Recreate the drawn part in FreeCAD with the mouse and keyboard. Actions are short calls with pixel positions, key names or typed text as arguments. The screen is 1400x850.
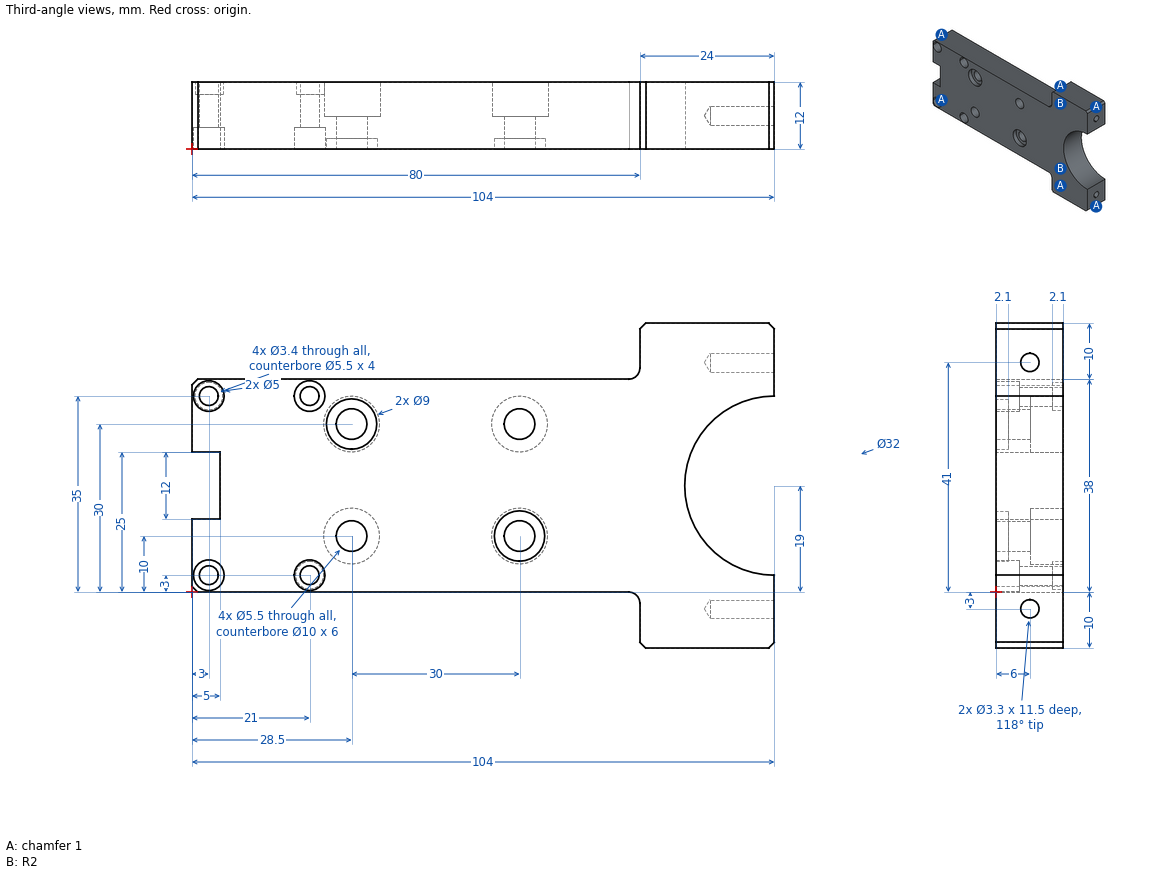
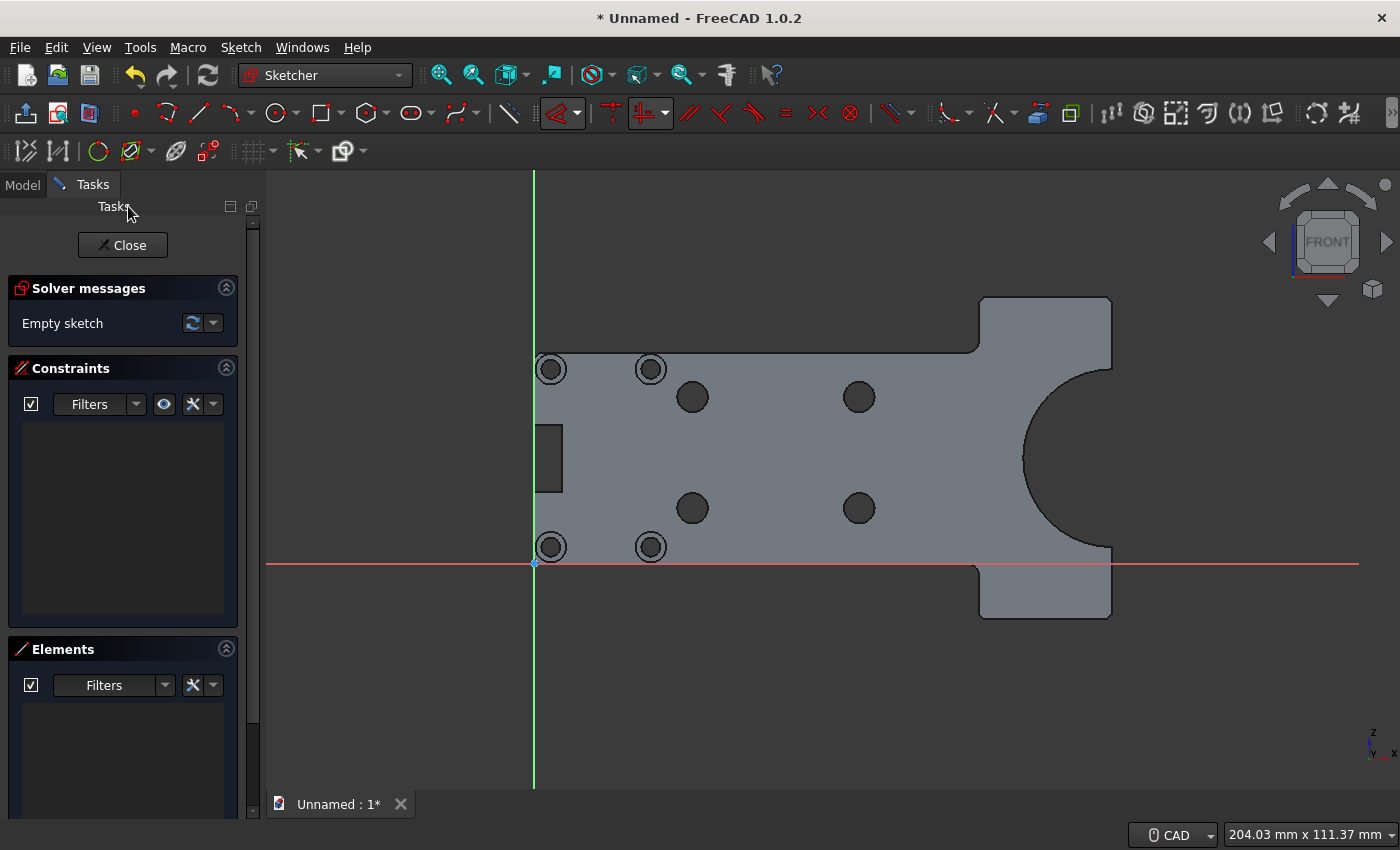
scroll(642, 454, up, 3)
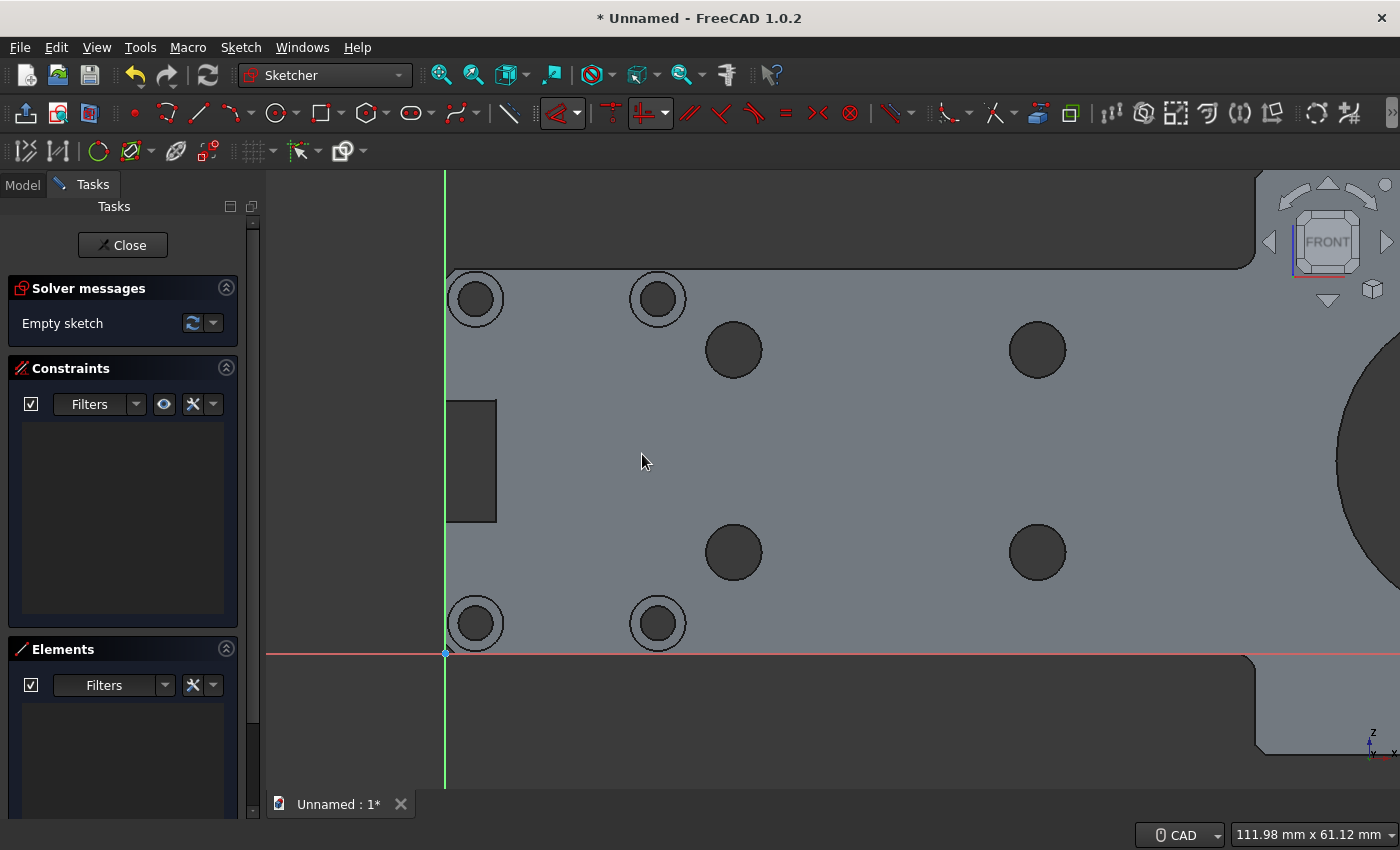
click(276, 114)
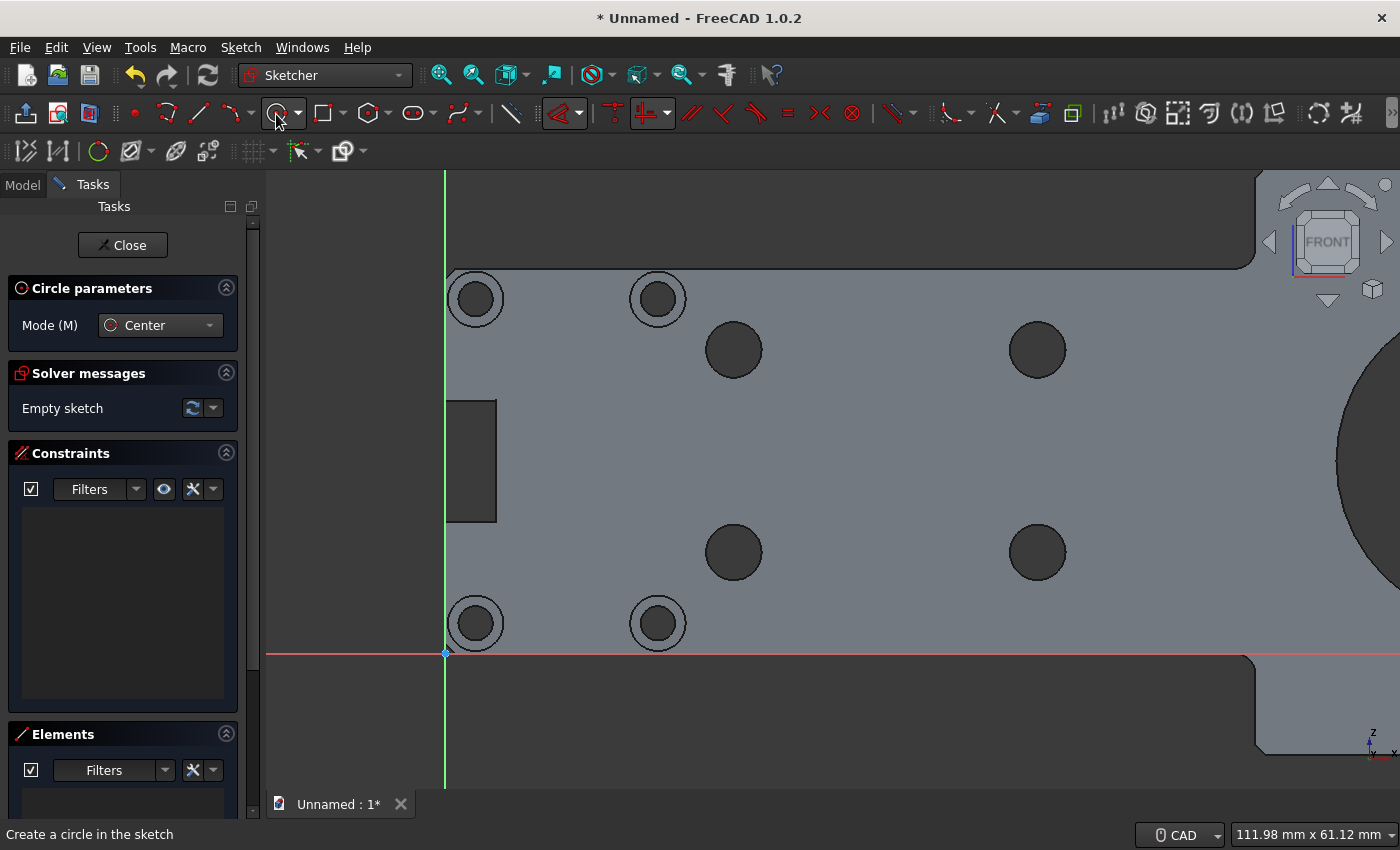
click(734, 350)
click(766, 318)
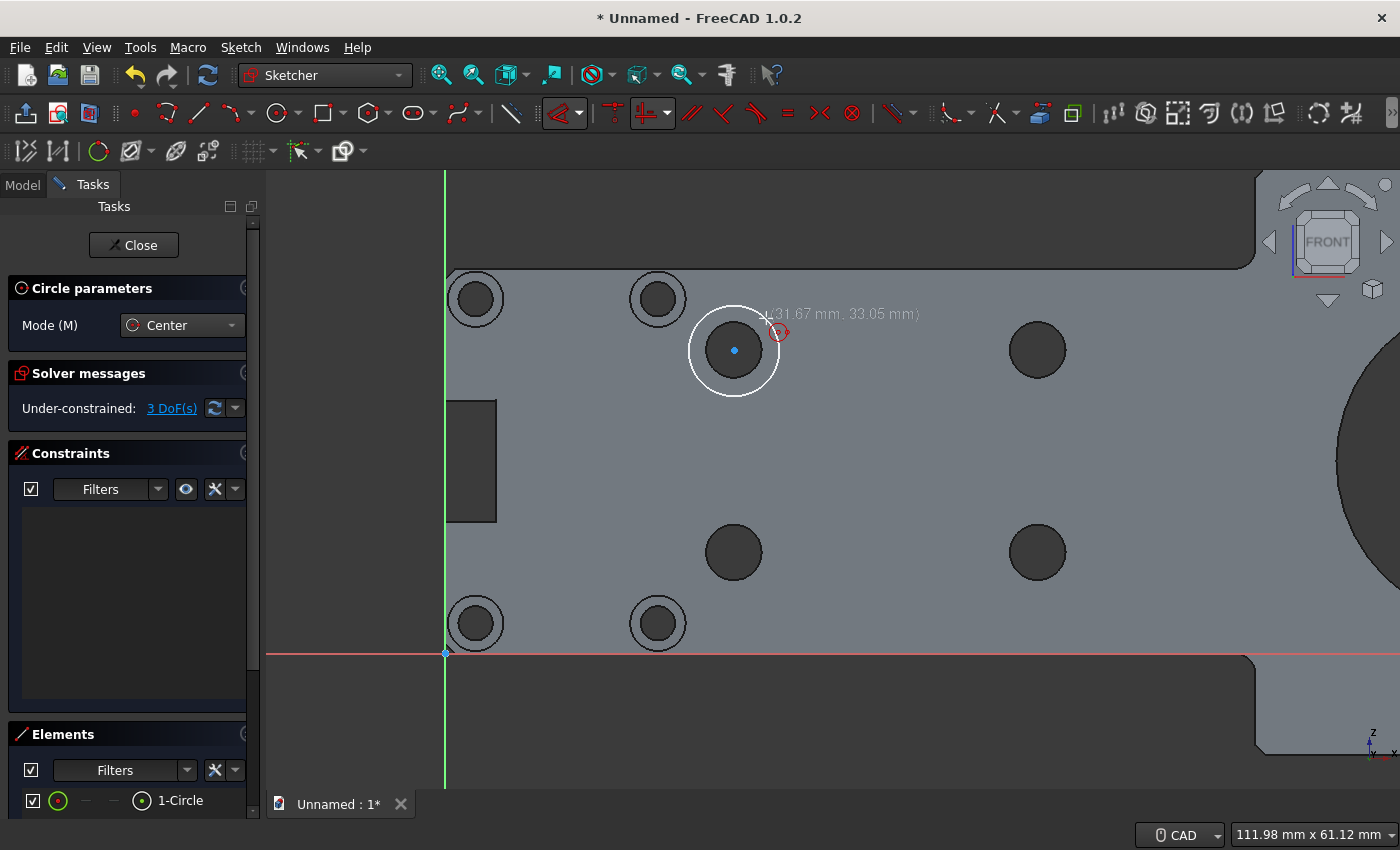
click(1038, 552)
click(1070, 520)
key(Escape)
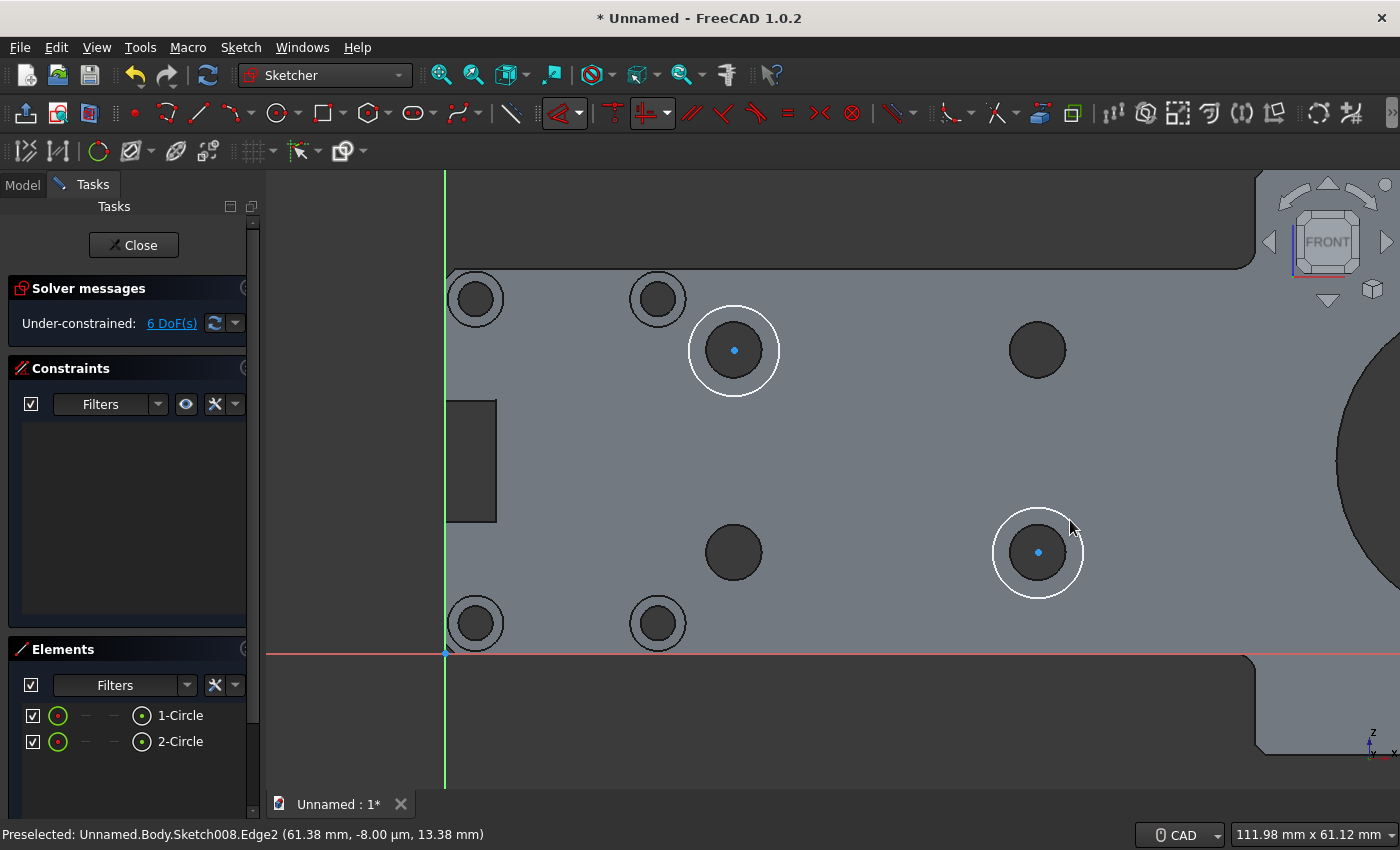
click(766, 319)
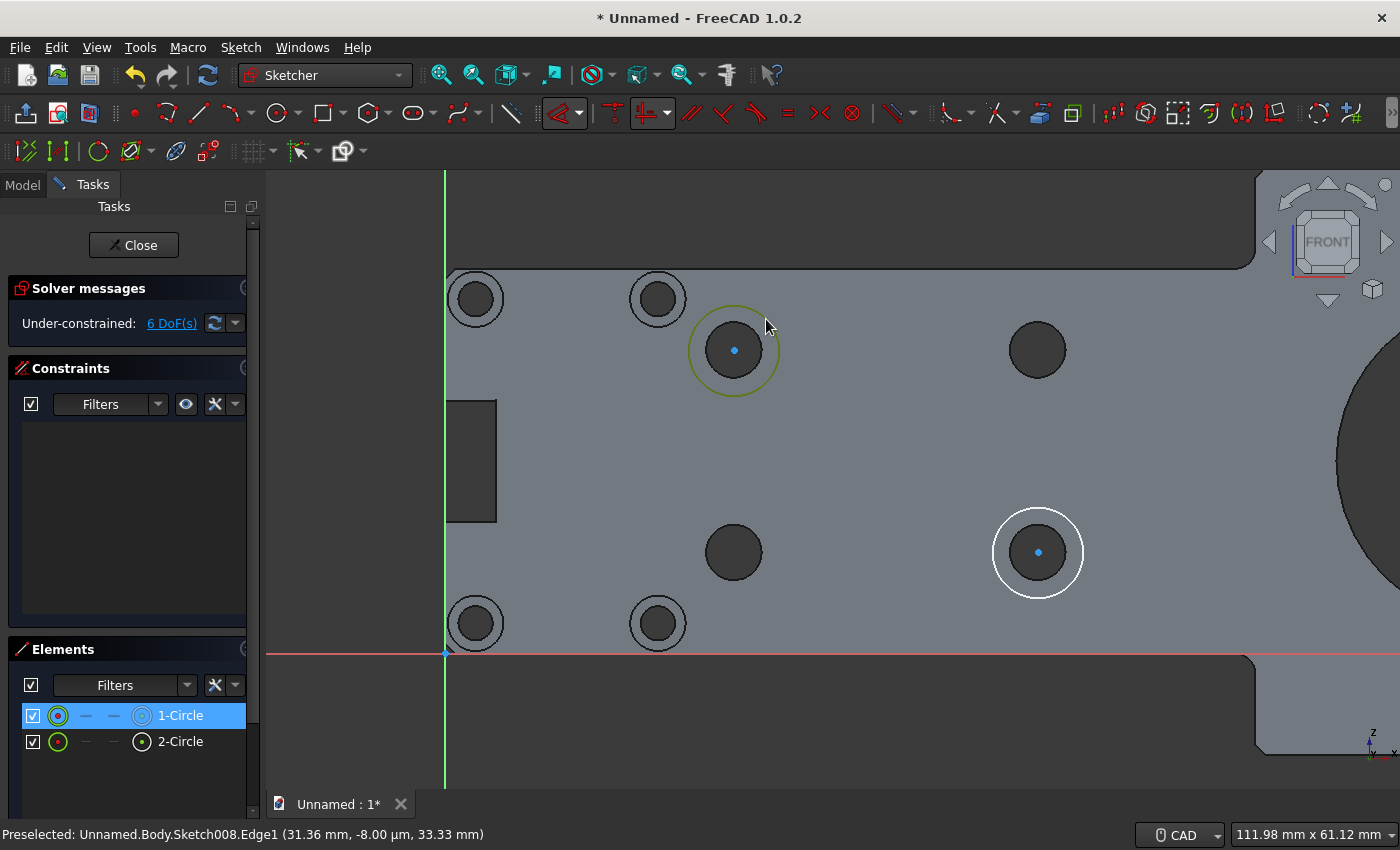
click(1070, 521)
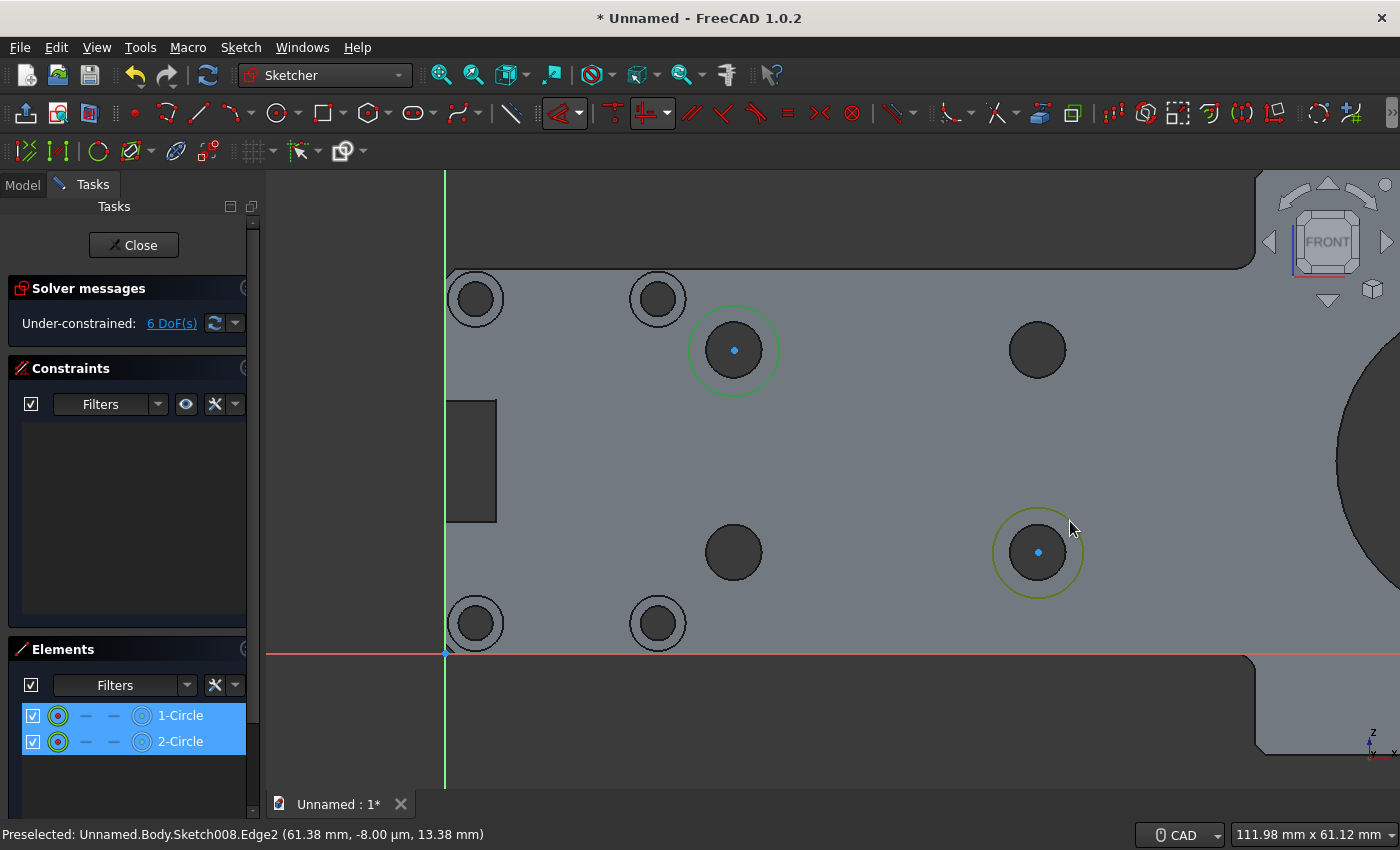
click(788, 114)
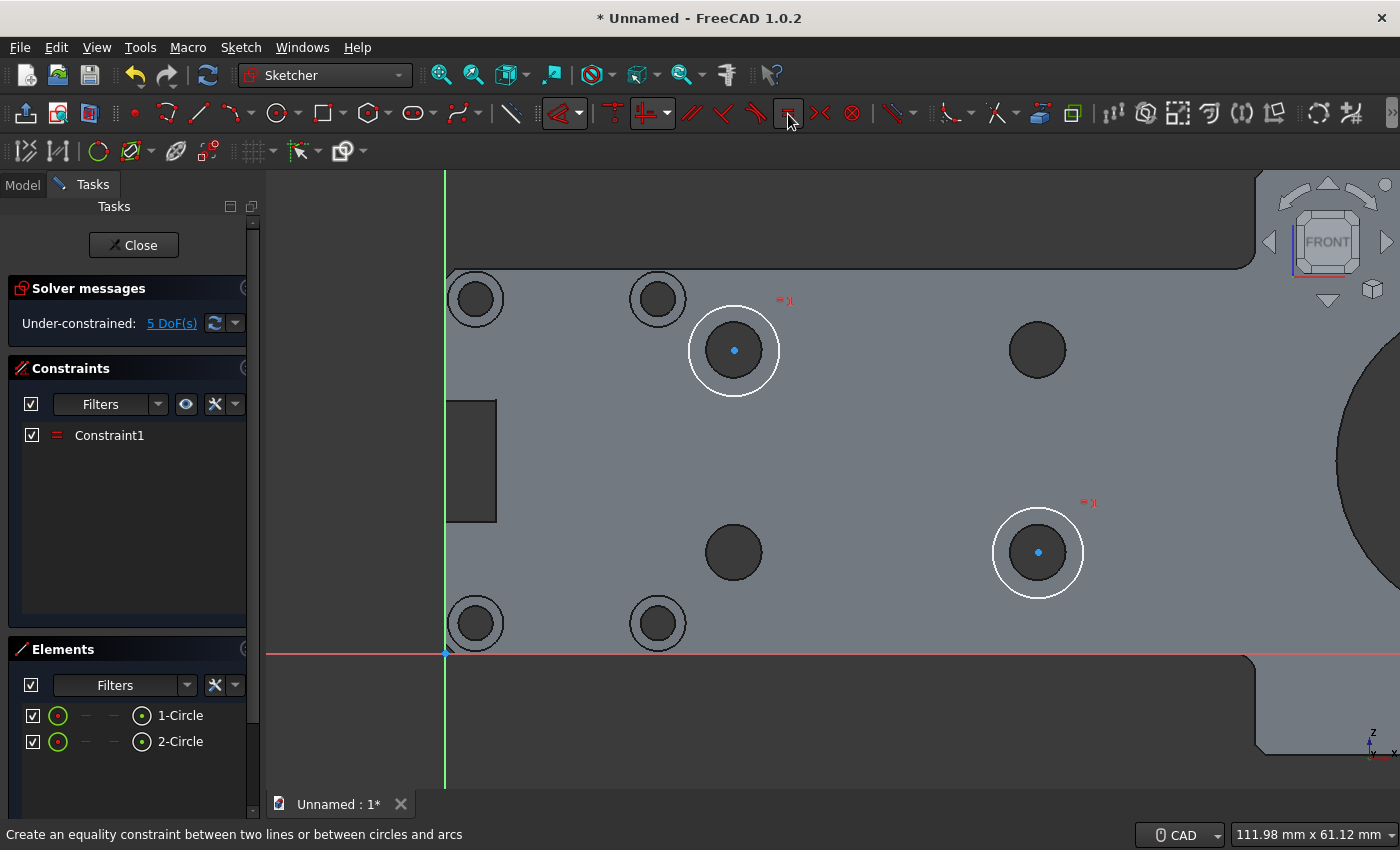
click(766, 319)